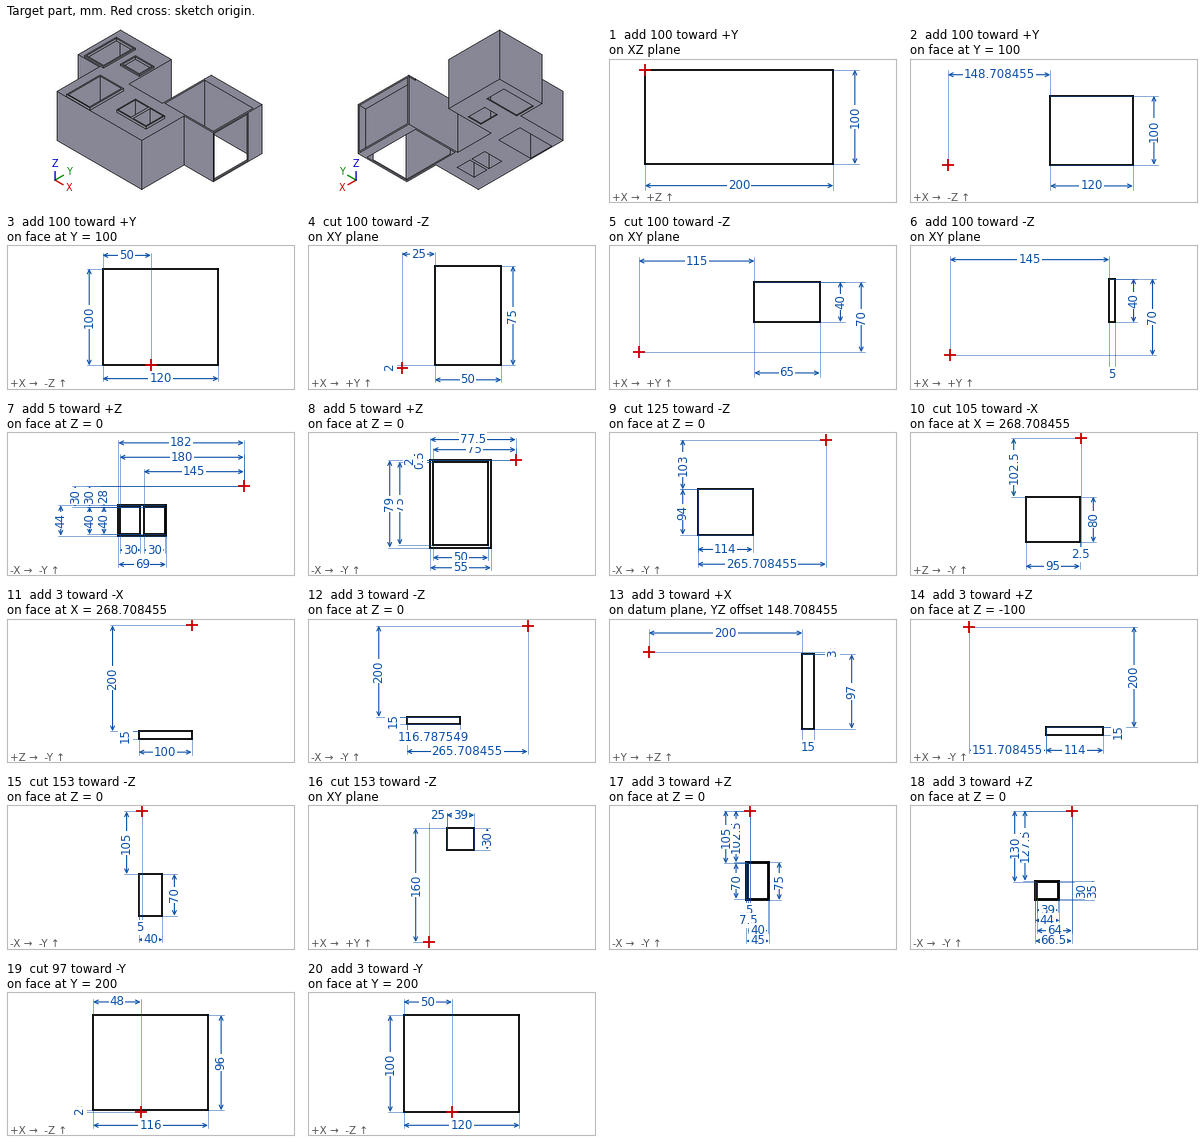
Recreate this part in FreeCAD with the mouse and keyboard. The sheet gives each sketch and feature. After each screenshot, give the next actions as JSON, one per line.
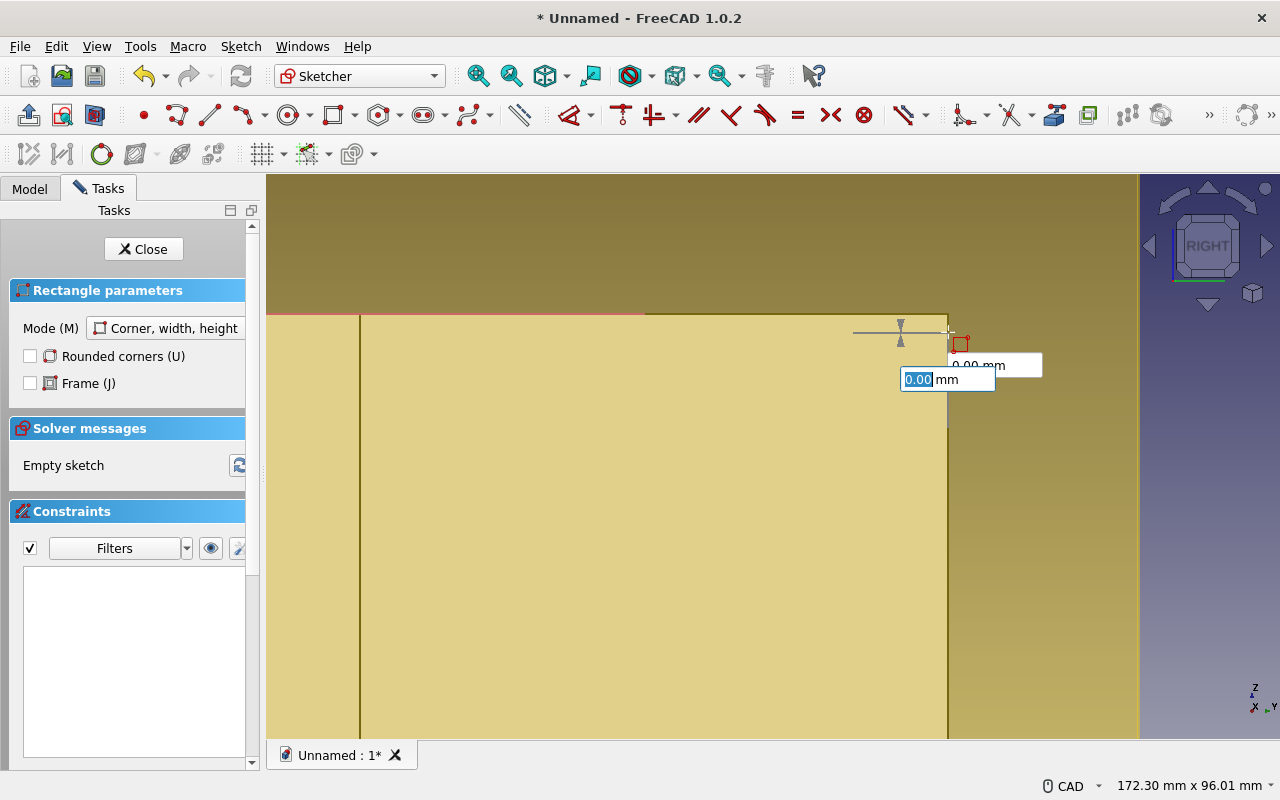
{"action": "scroll", "coordinate": [950, 333], "scroll_direction": "down", "scroll_amount": 4}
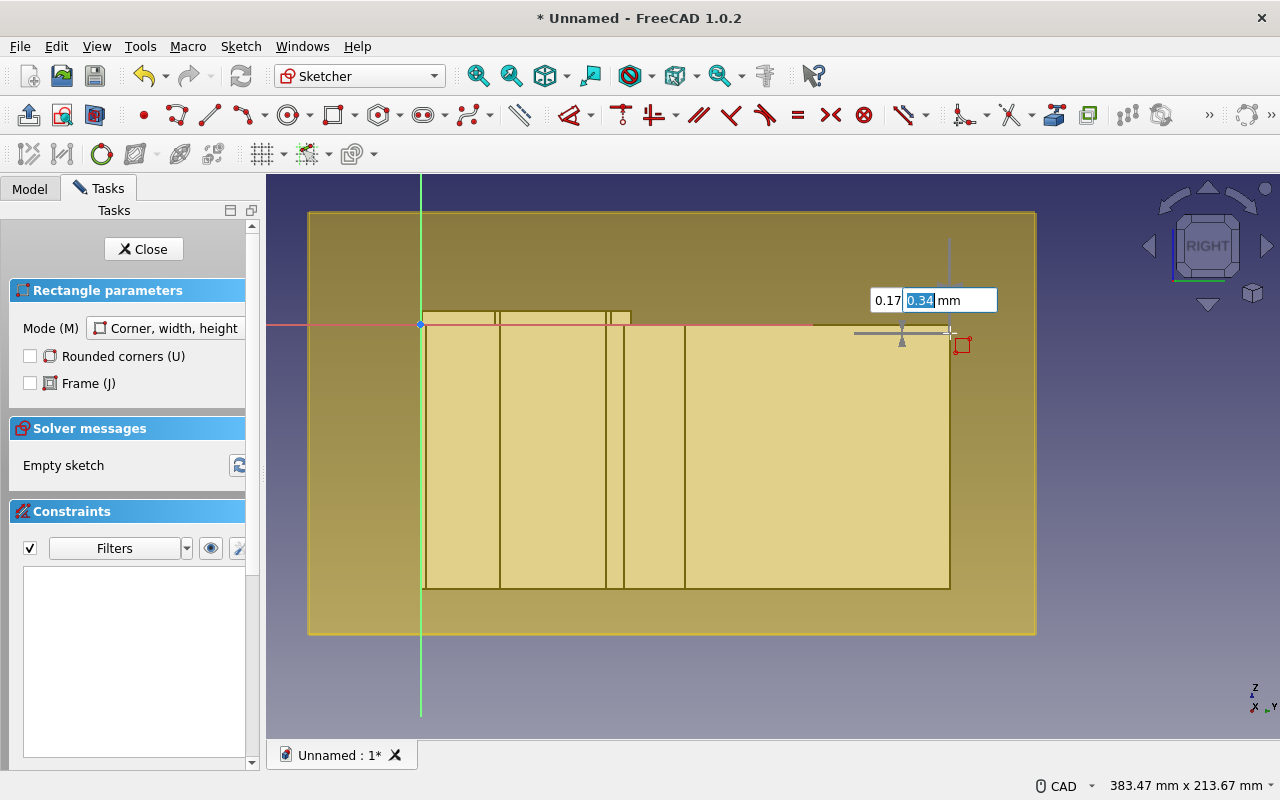
{"action": "left_click", "coordinate": [989, 589]}
{"action": "key", "text": "Escape"}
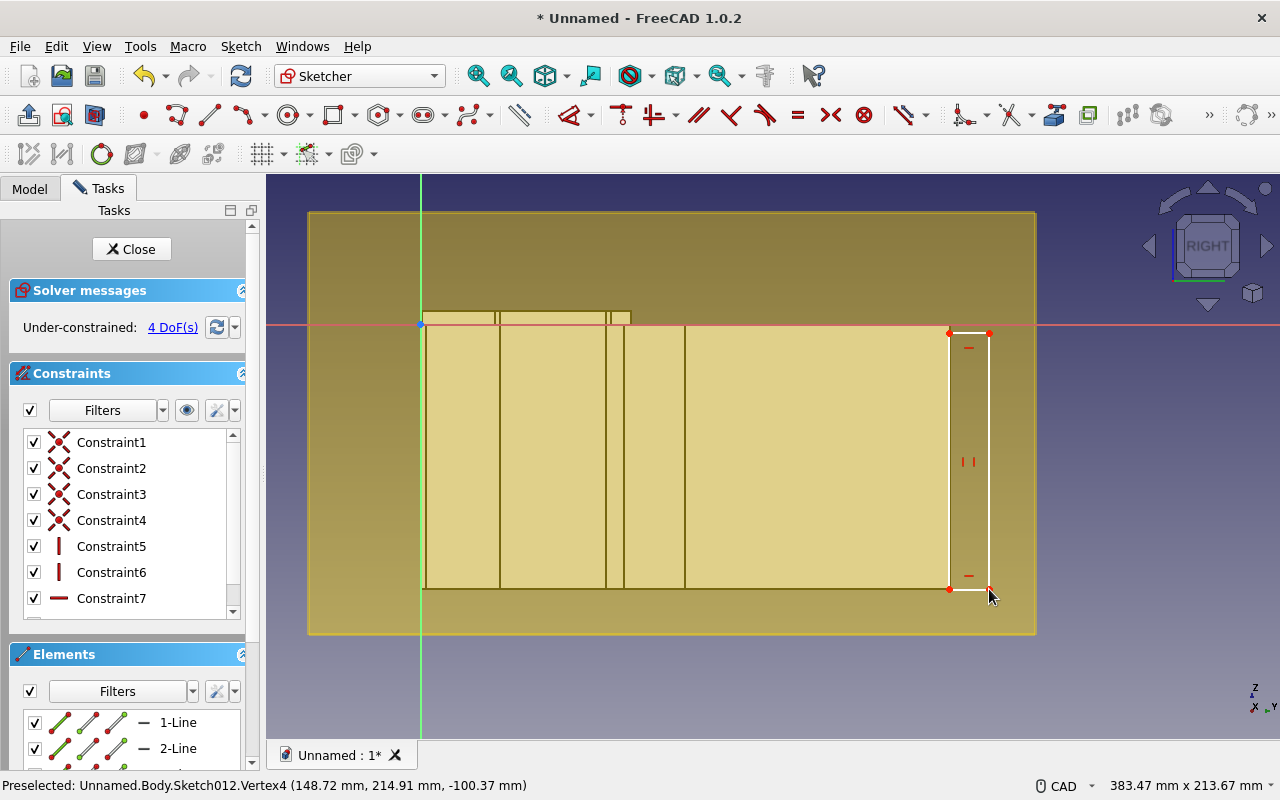
{"action": "left_click", "coordinate": [568, 116]}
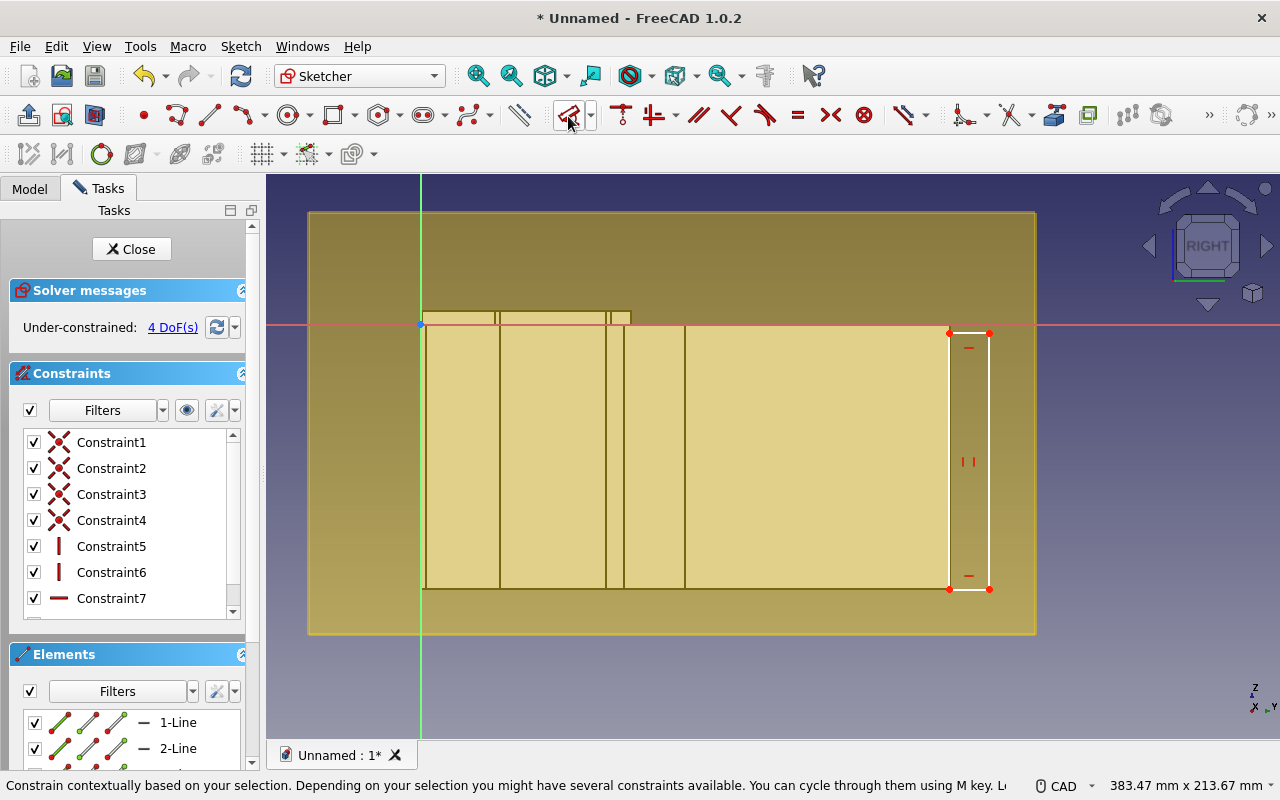
{"action": "left_click", "coordinate": [949, 410]}
{"action": "left_click", "coordinate": [915, 462]}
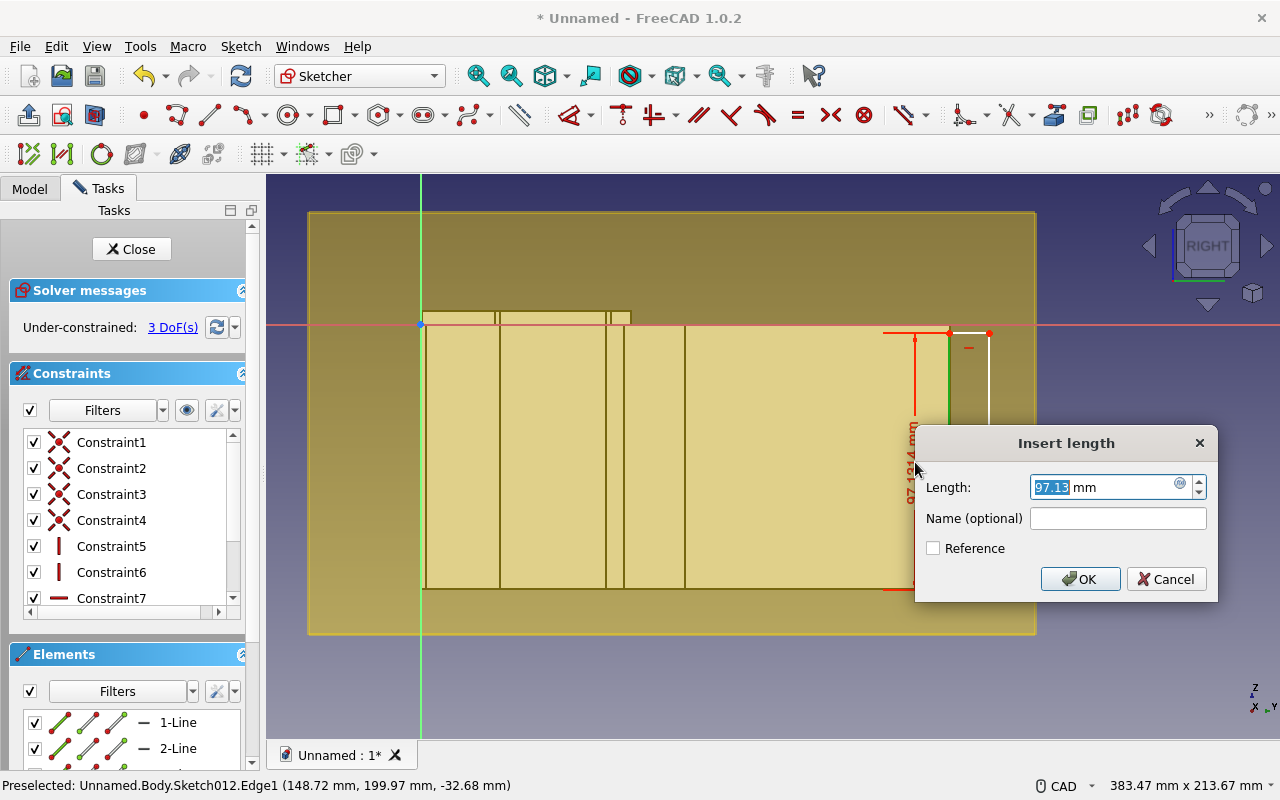
{"action": "type", "text": "97"}
{"action": "key", "text": "Return"}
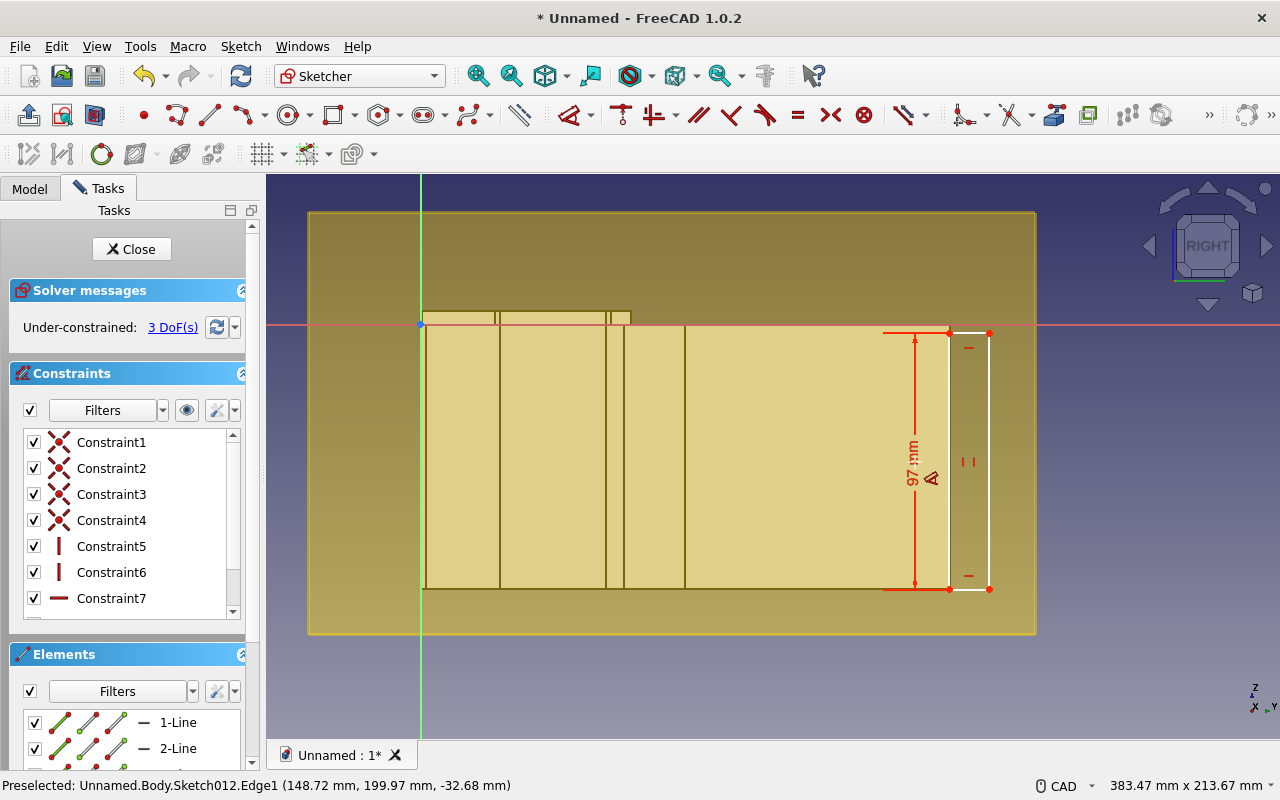
{"action": "left_click", "coordinate": [961, 590]}
{"action": "left_click", "coordinate": [969, 624]}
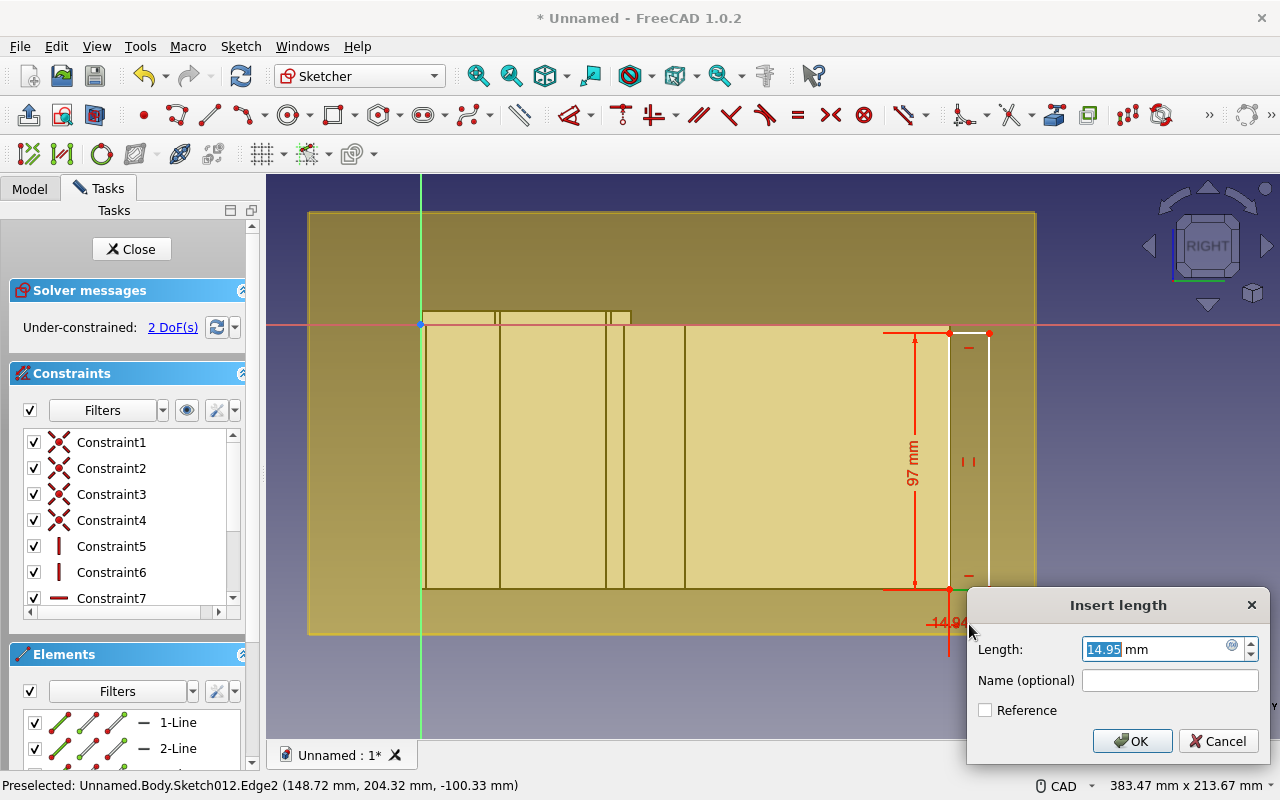
{"action": "type", "text": "15"}
{"action": "key", "text": "Return"}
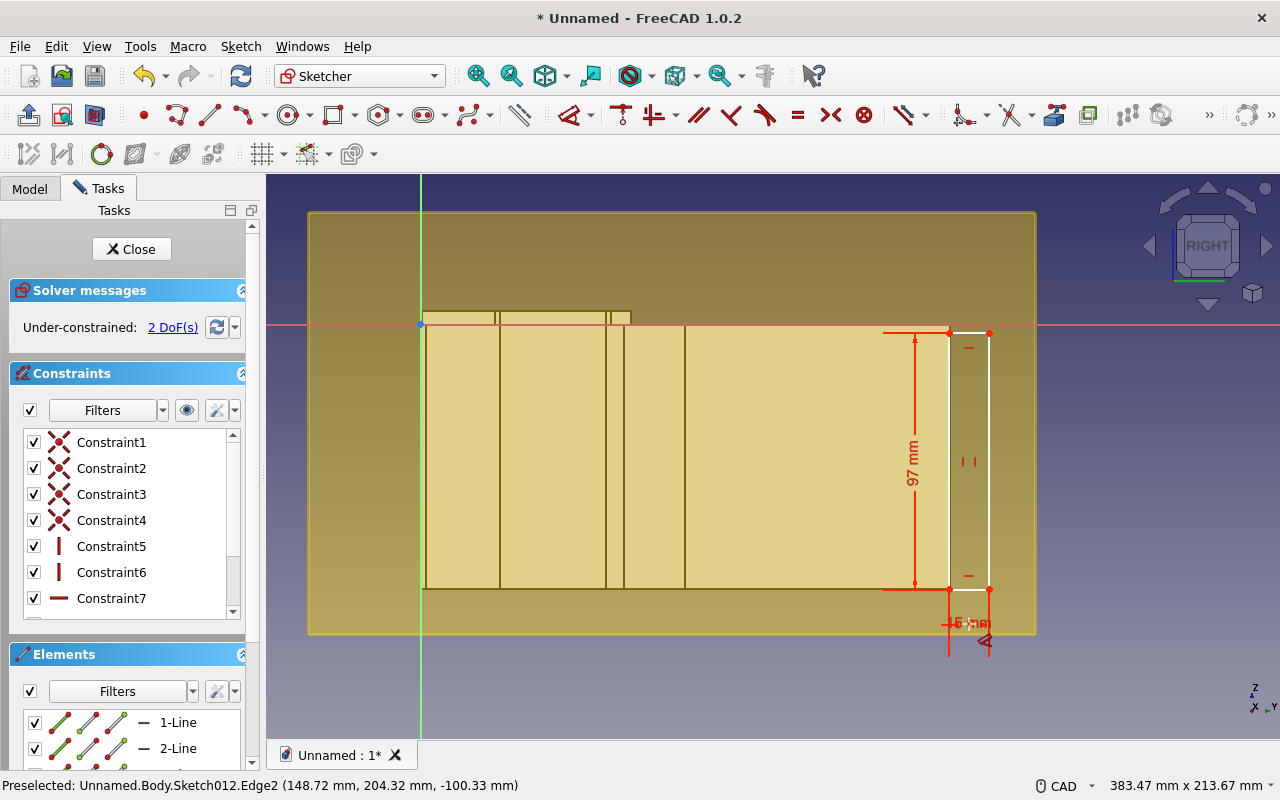
{"action": "scroll", "coordinate": [949, 333], "scroll_direction": "up", "scroll_amount": 9}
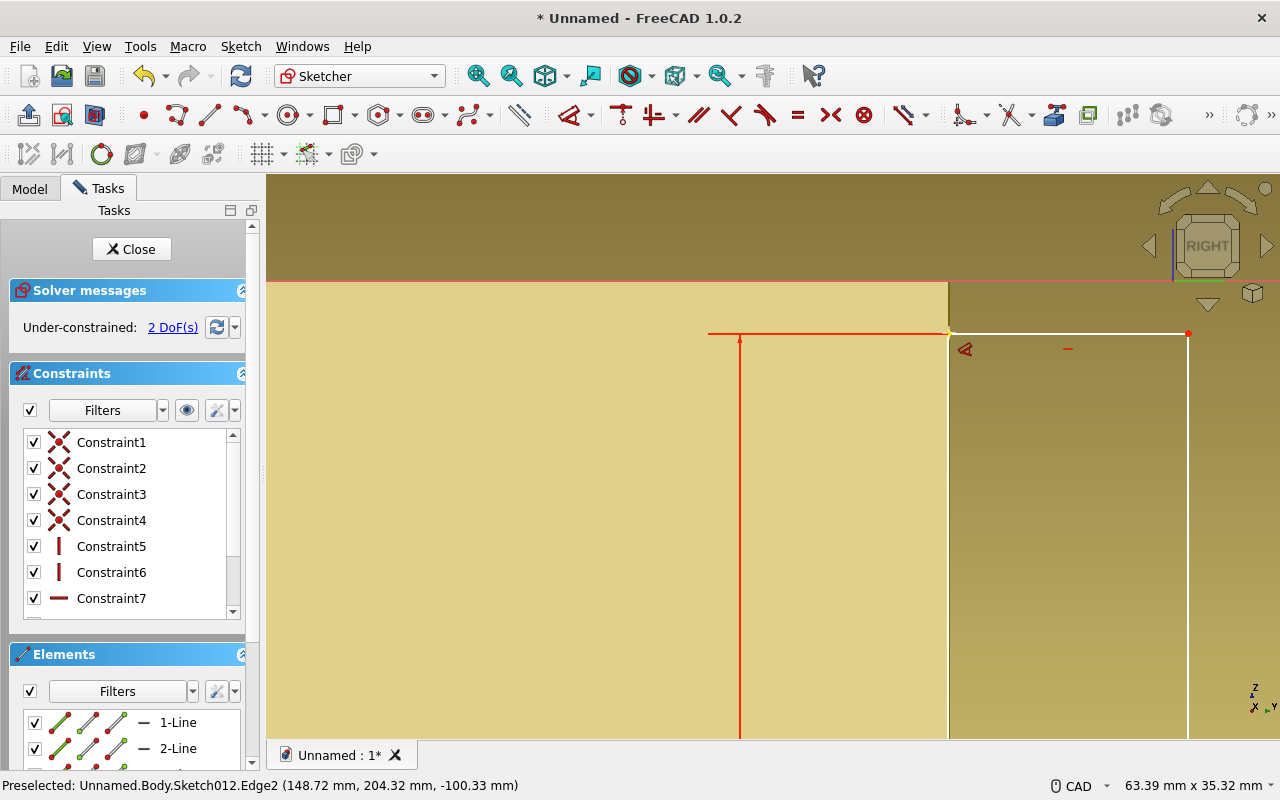
{"action": "left_click", "coordinate": [948, 334]}
{"action": "left_click", "coordinate": [982, 307]}